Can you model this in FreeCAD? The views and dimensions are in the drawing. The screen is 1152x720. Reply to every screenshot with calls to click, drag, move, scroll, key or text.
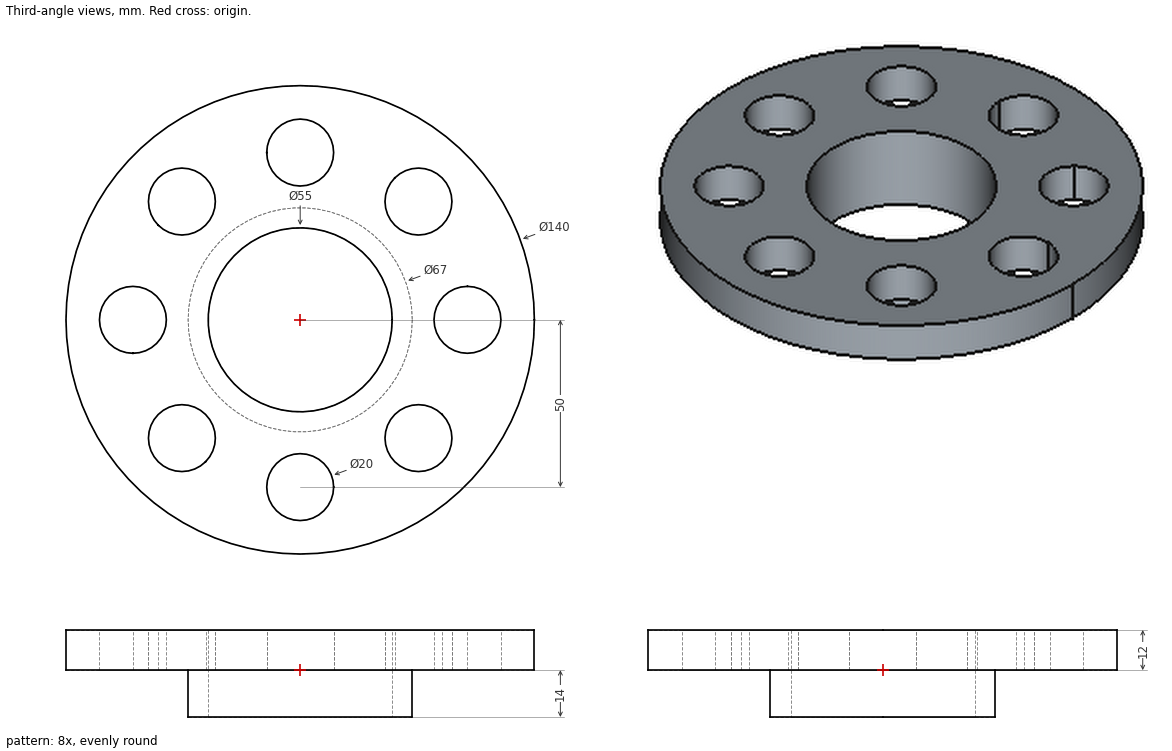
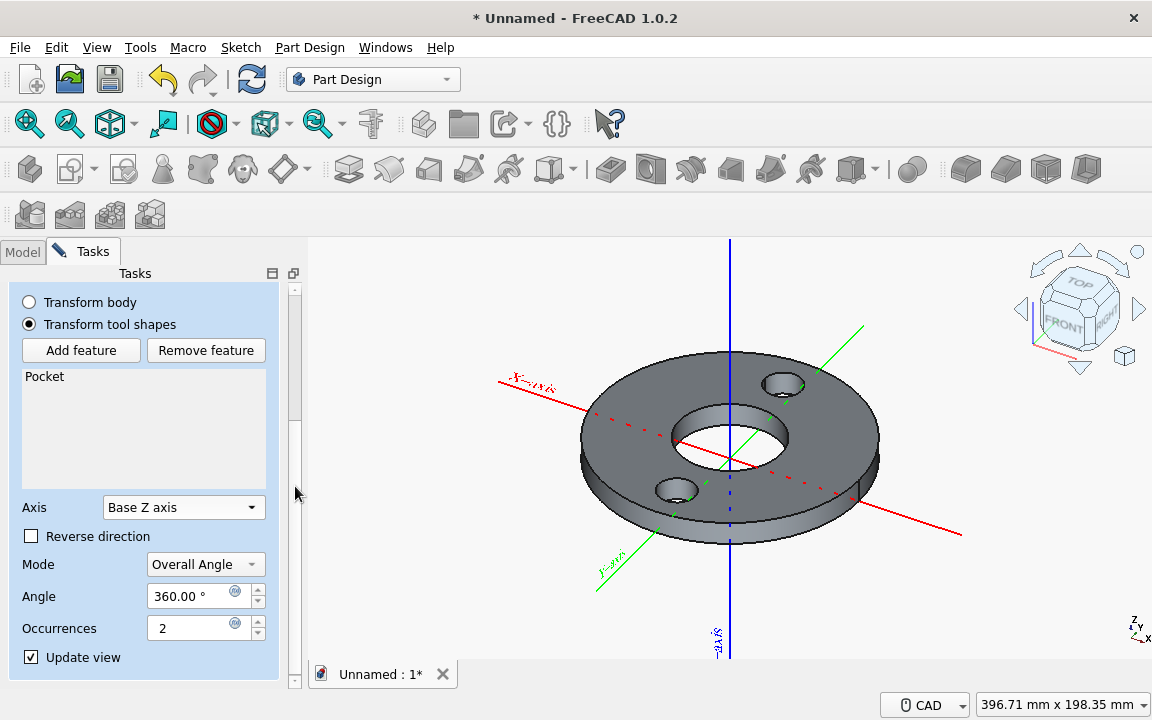
triple_click(198, 628)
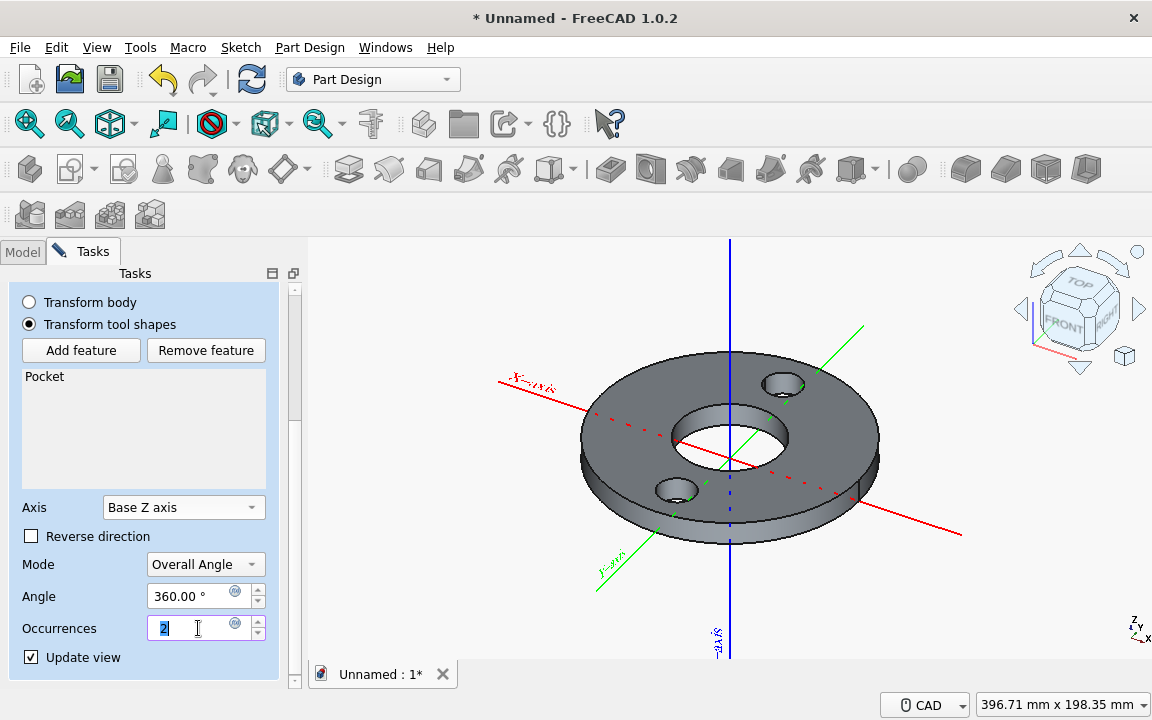
text(8)
key(Tab)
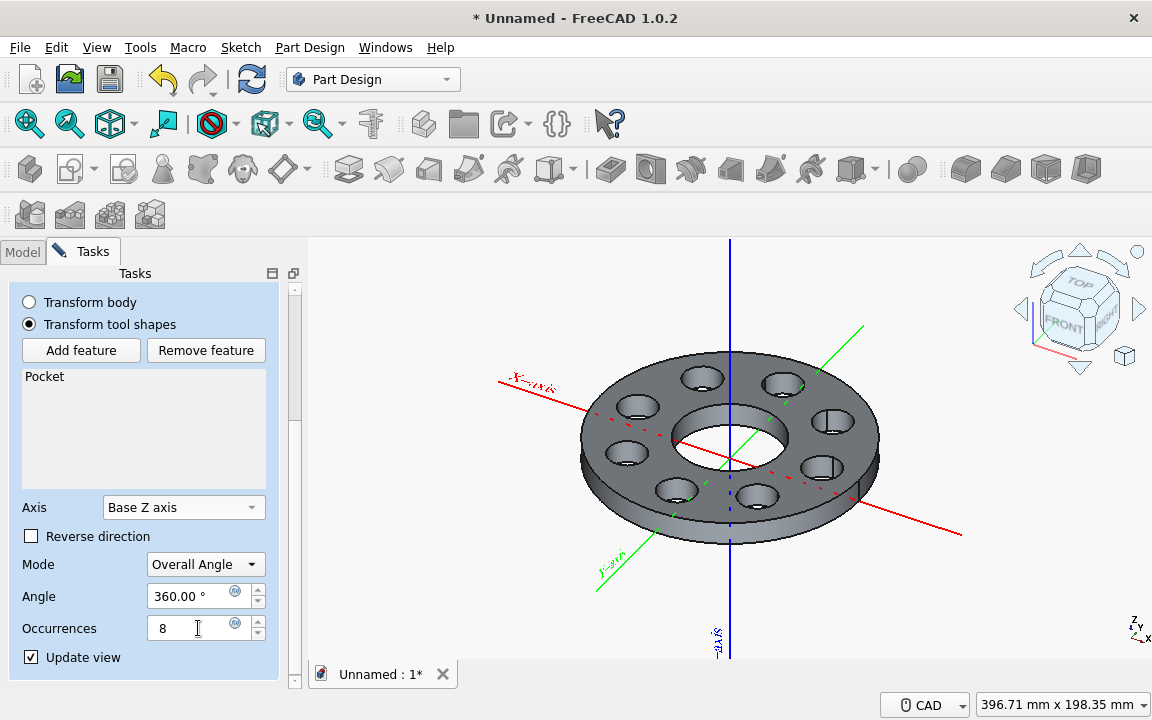
scroll(295, 486, up, 5)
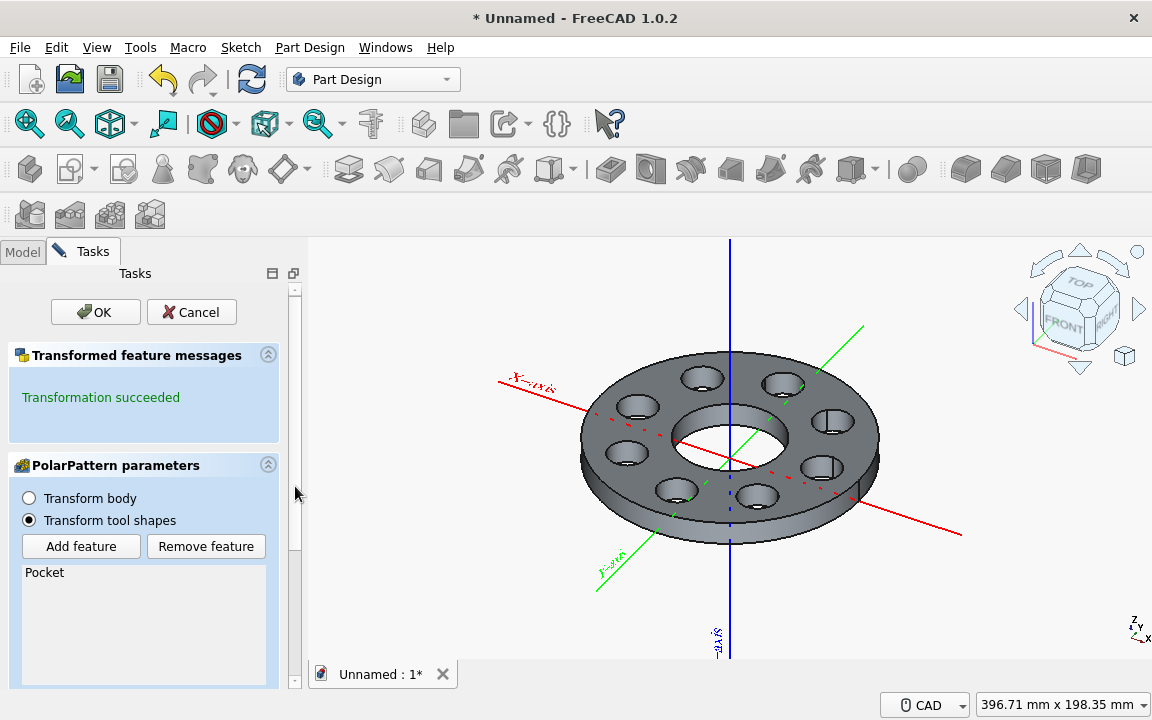
click(96, 312)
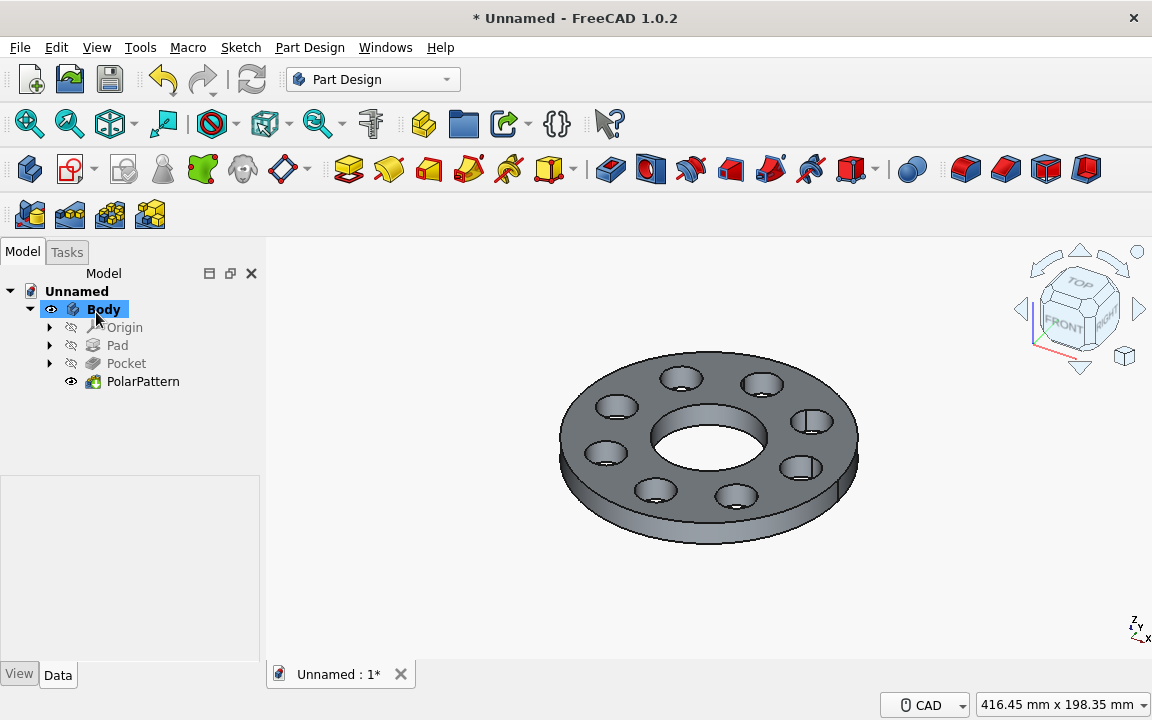
click(50, 327)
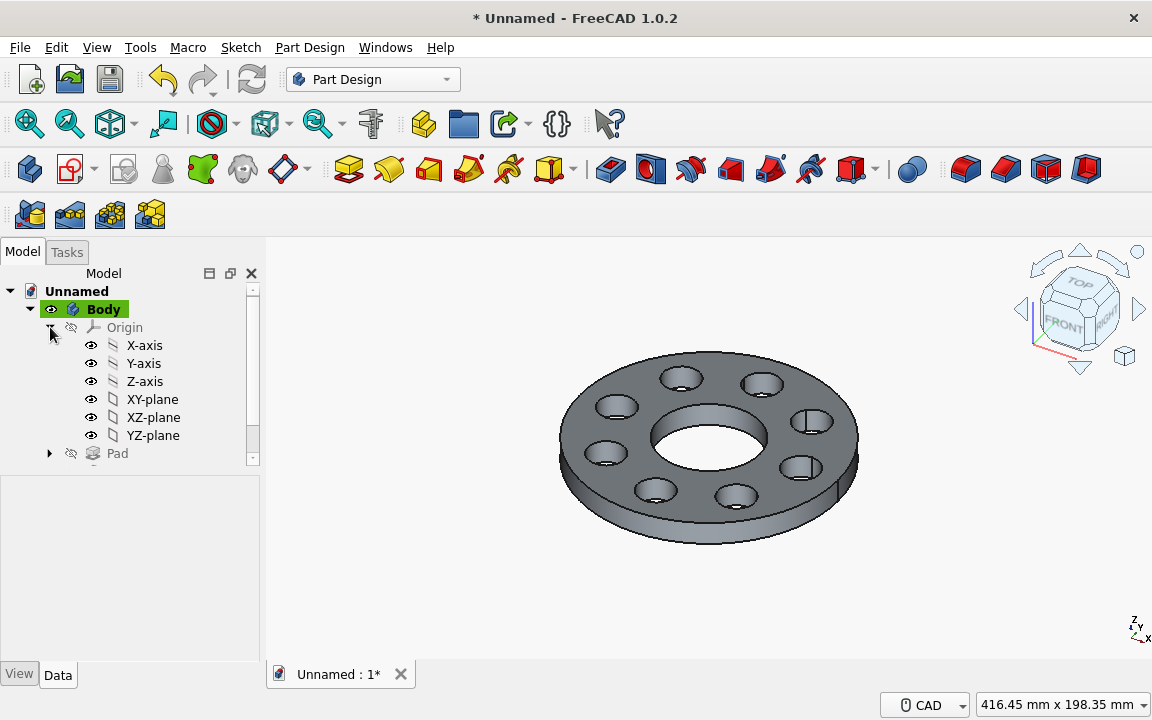
click(136, 399)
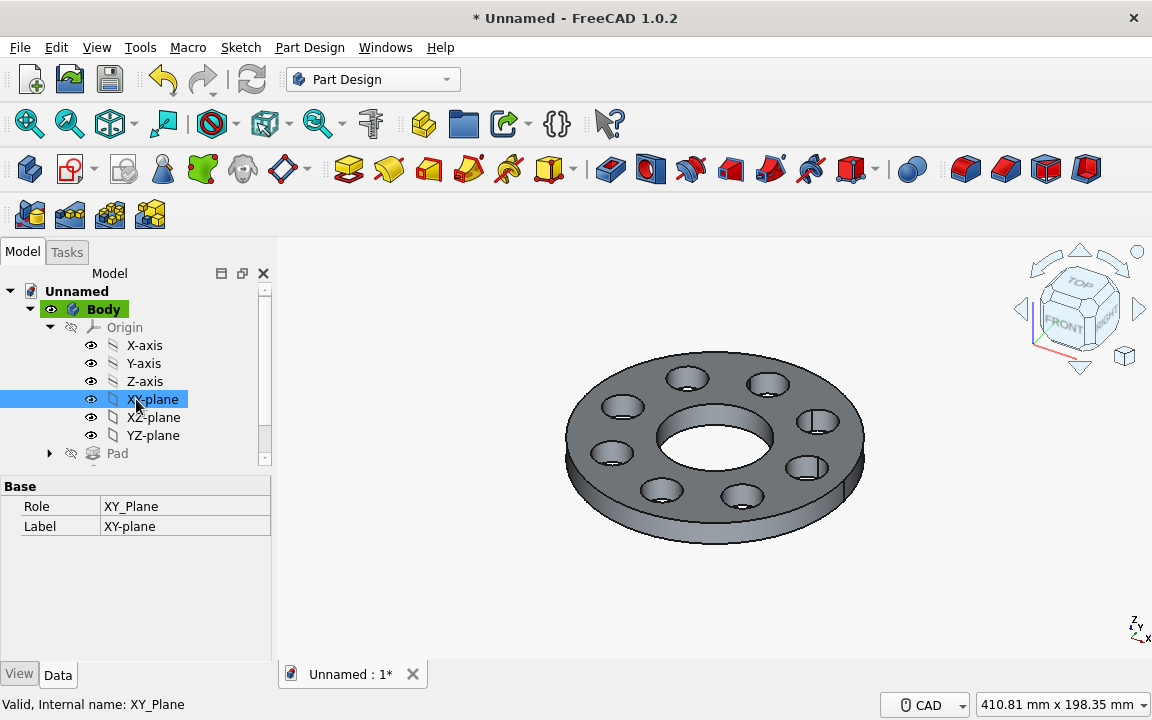
click(284, 170)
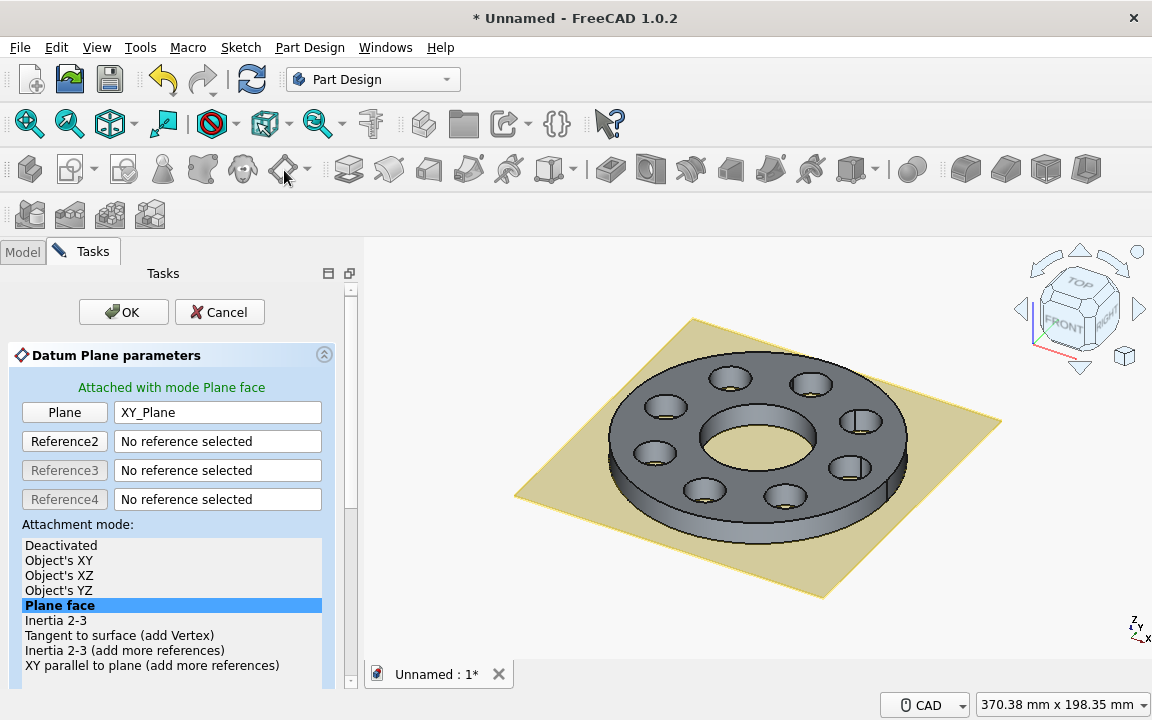
scroll(351, 486, down, 4)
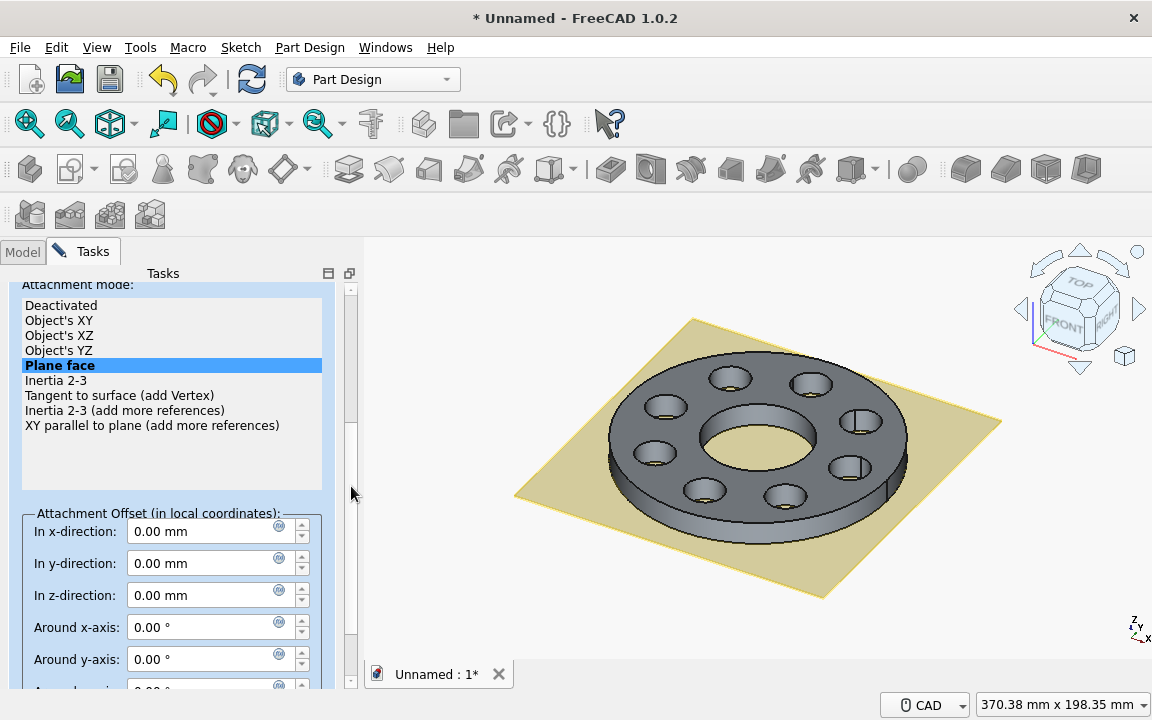
triple_click(210, 595)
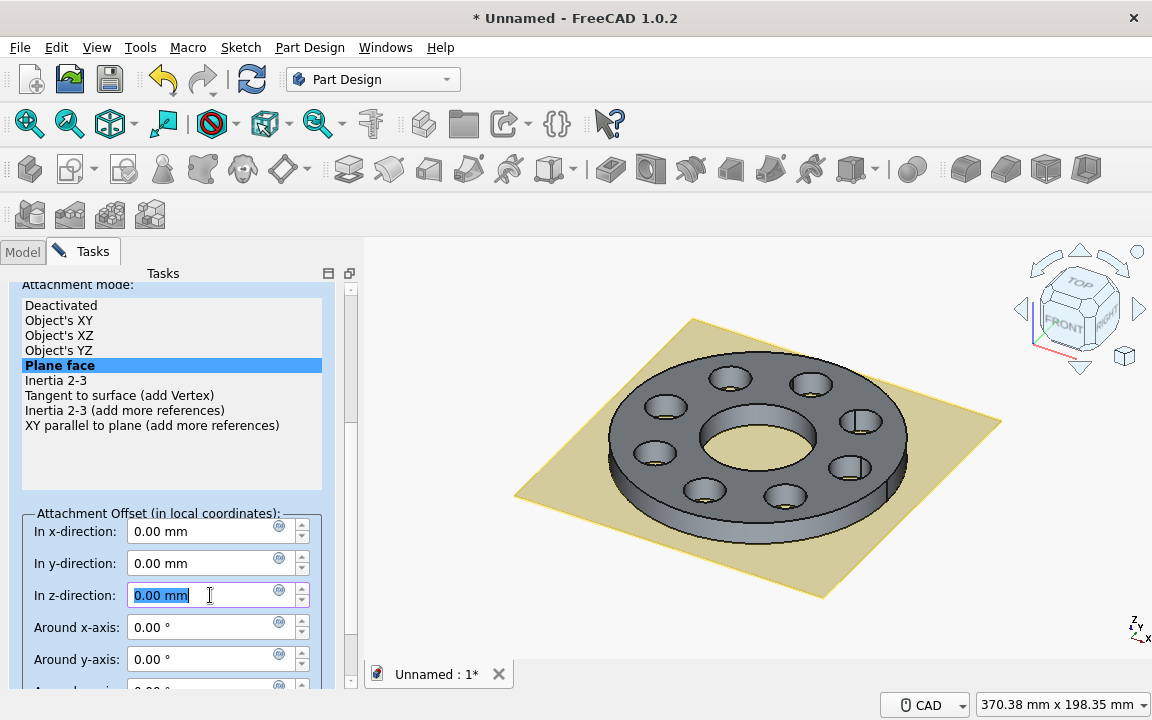
text(-14)
key(Tab)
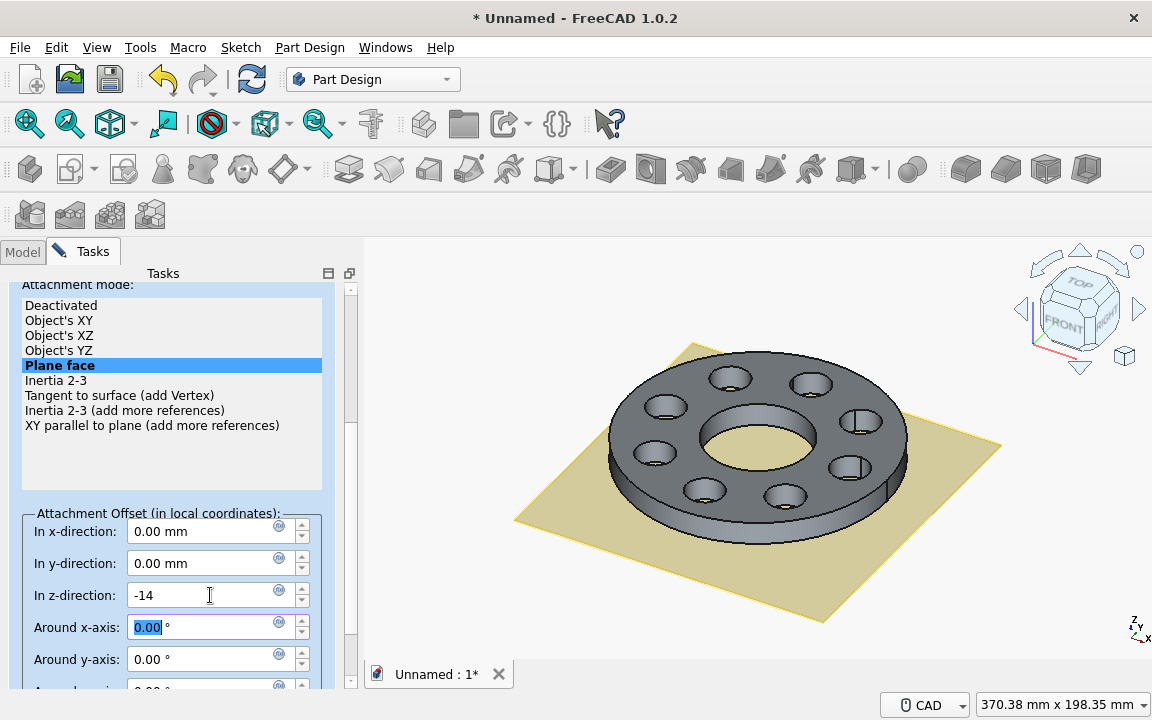
scroll(351, 486, up, 5)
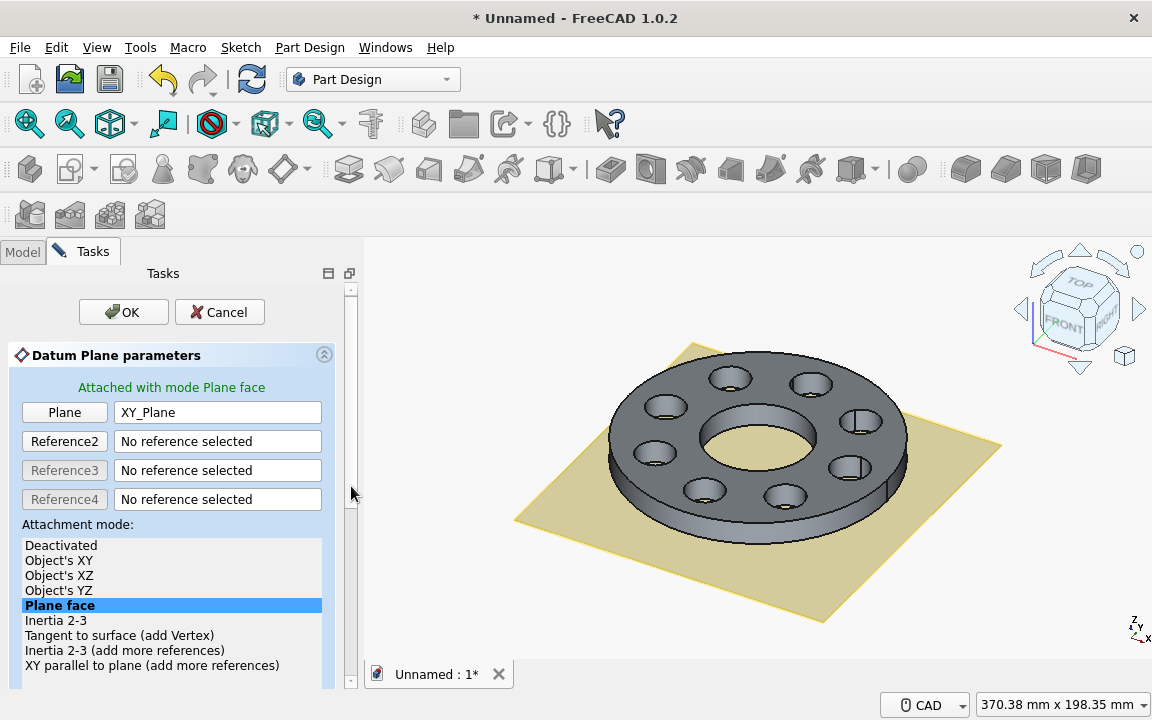
click(124, 312)